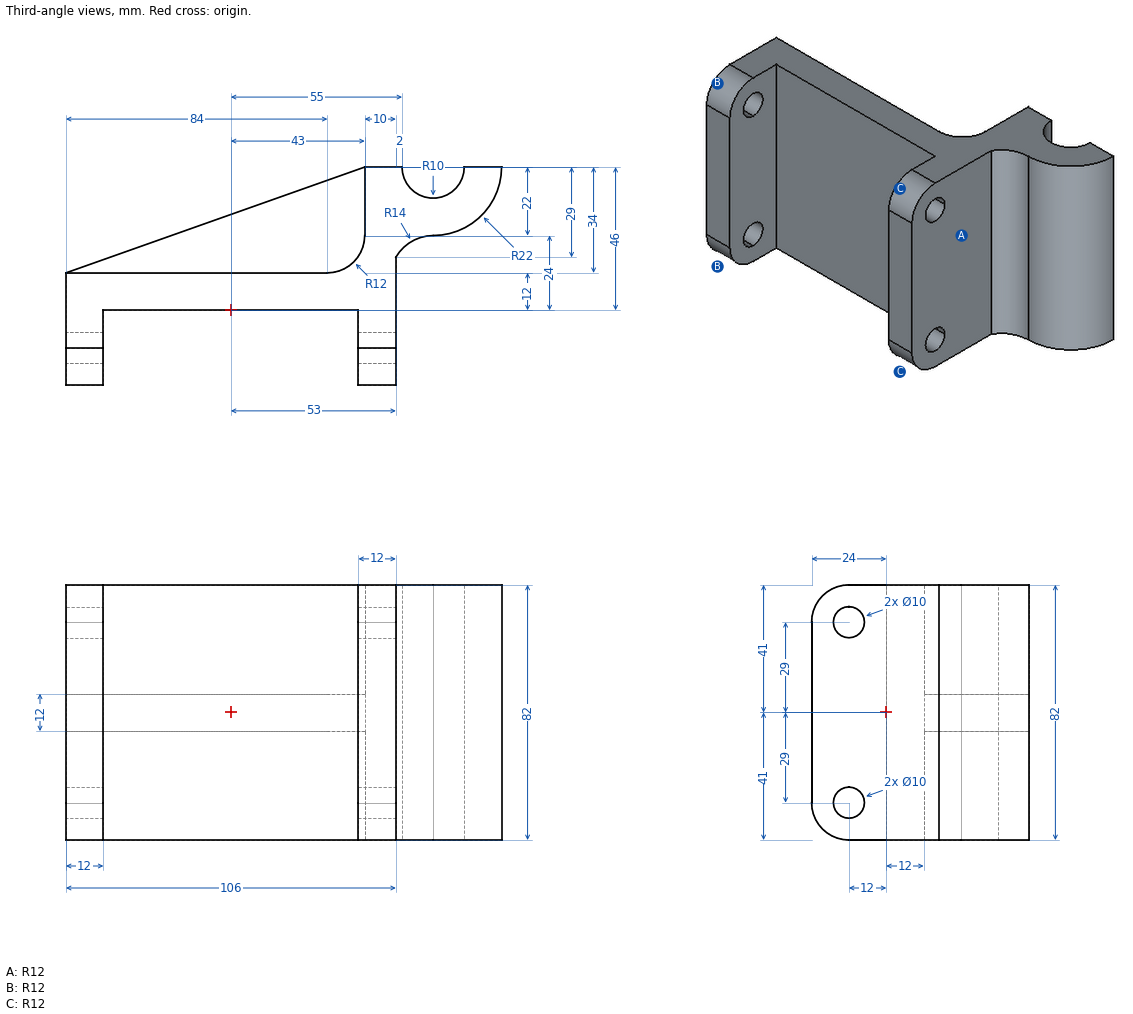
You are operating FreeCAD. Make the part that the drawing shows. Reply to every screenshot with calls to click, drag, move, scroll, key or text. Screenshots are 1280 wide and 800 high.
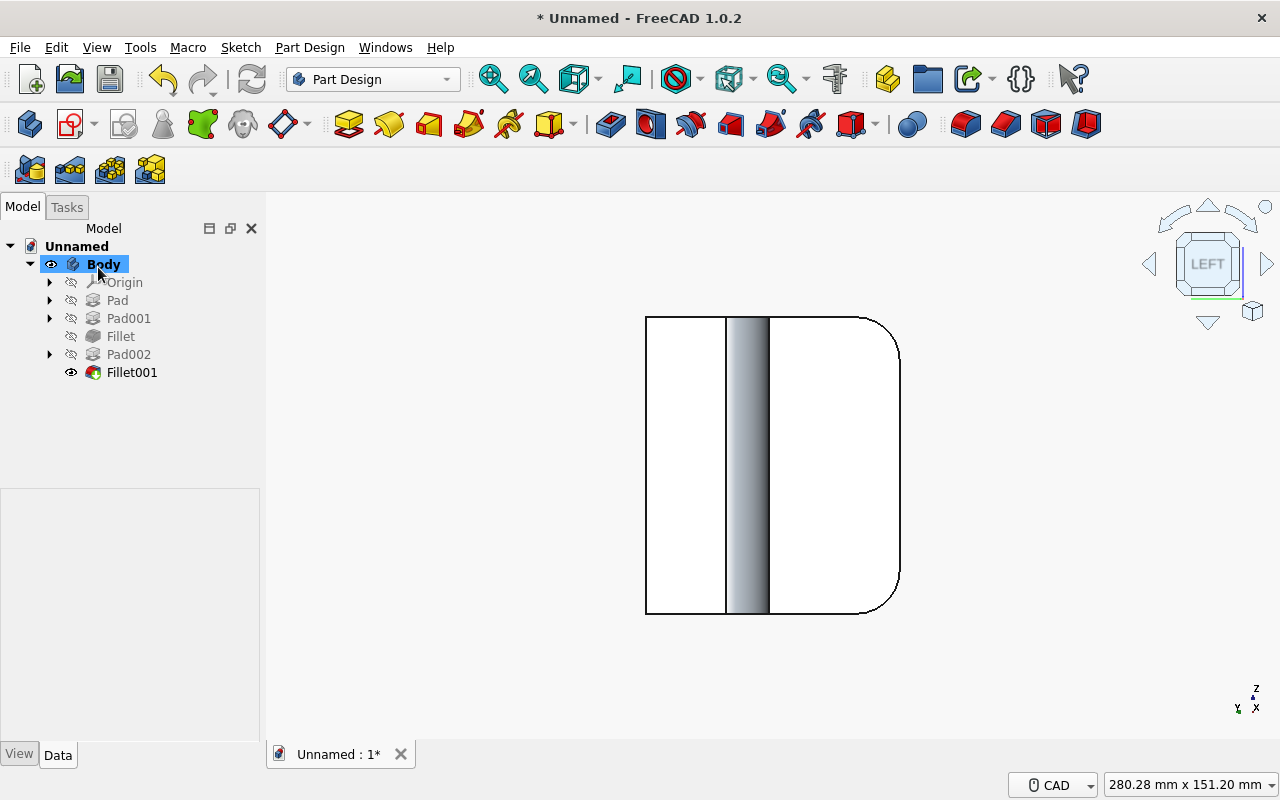
click(835, 422)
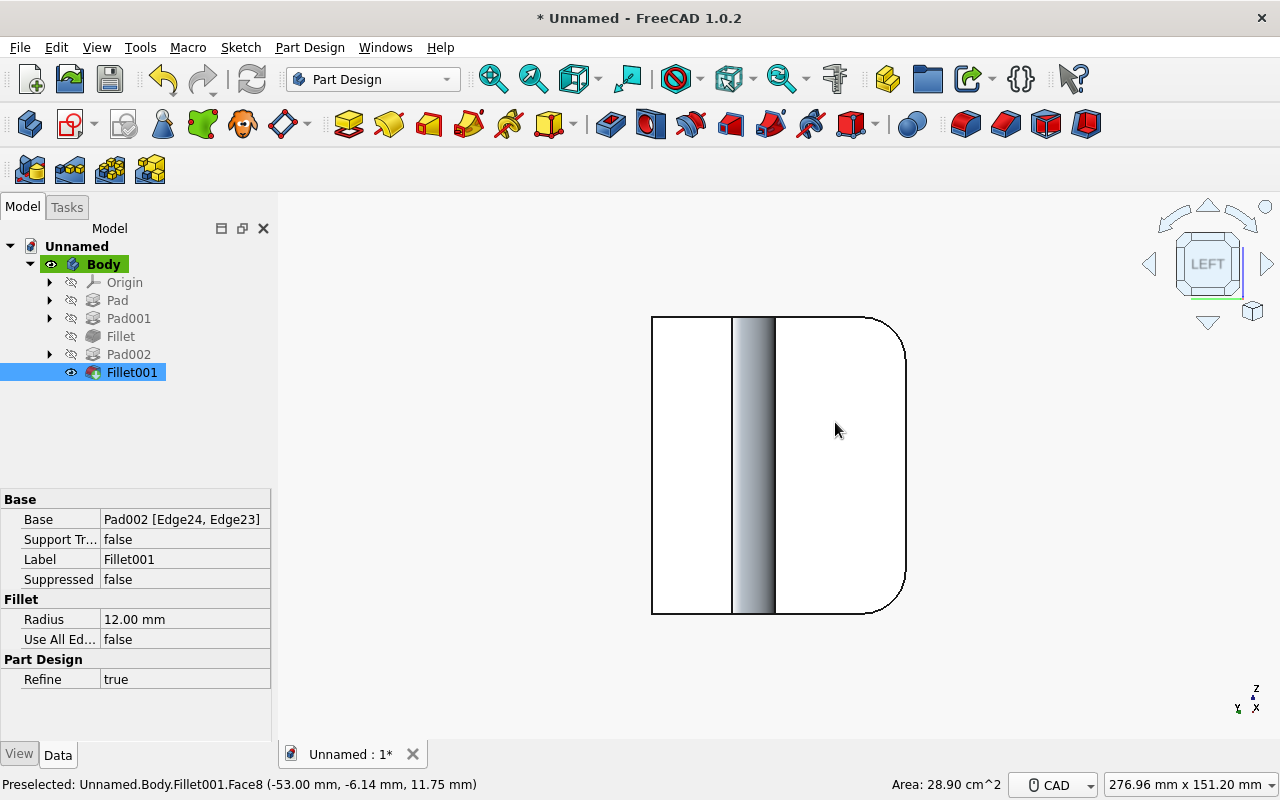
click(70, 124)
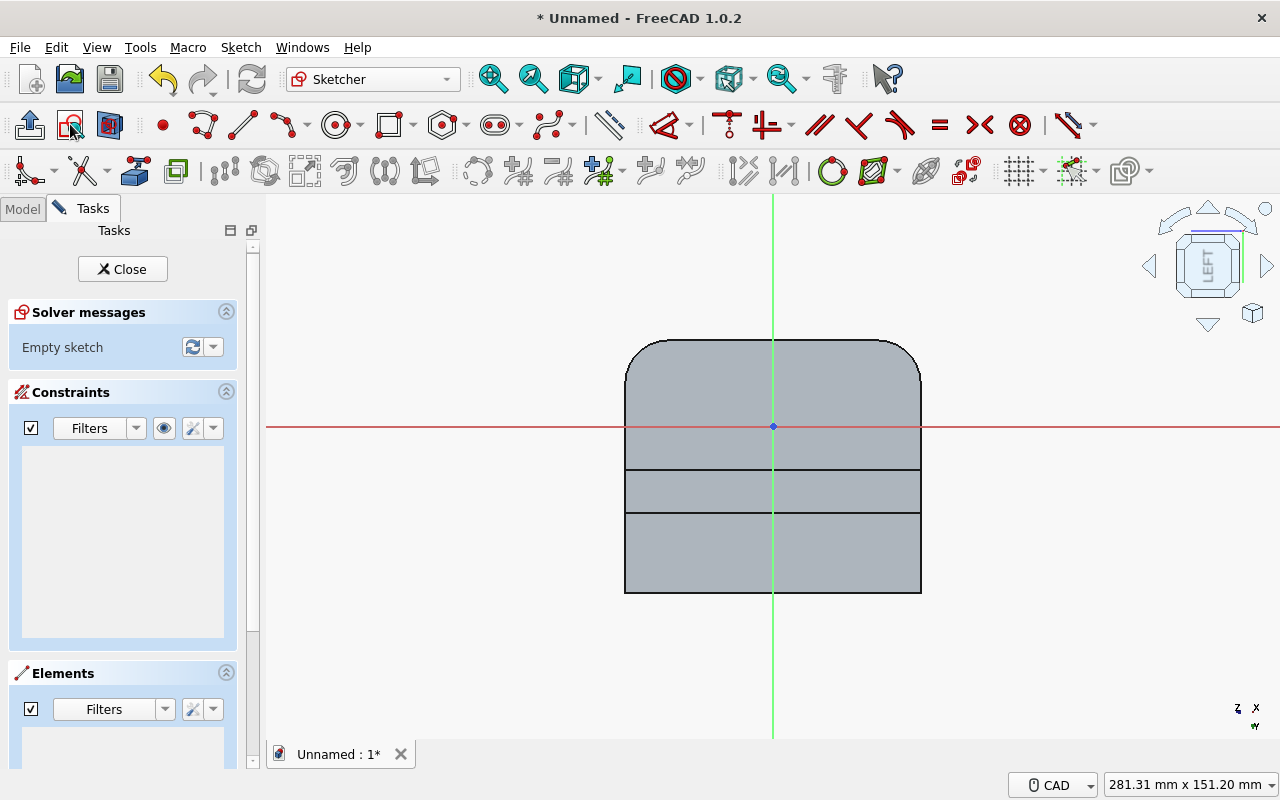
scroll(829, 339, up, 4)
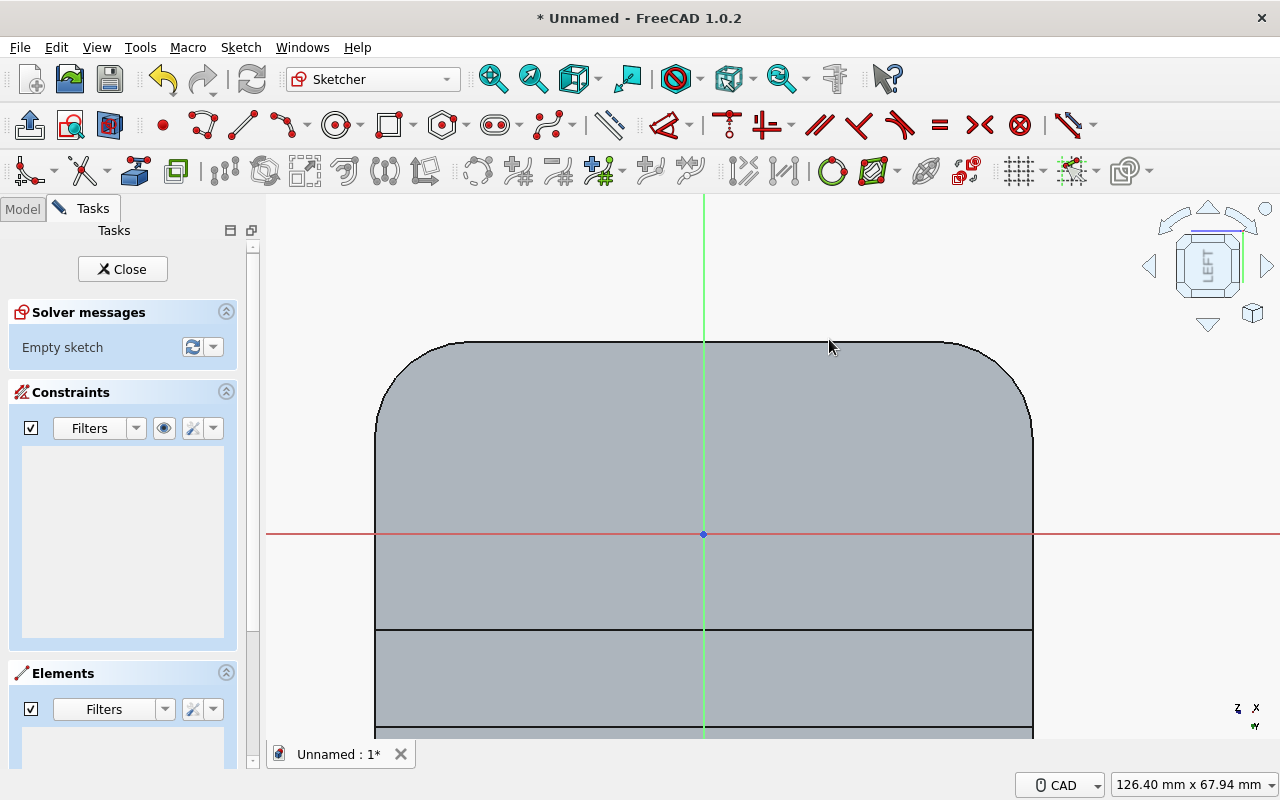
key(g)
key(c)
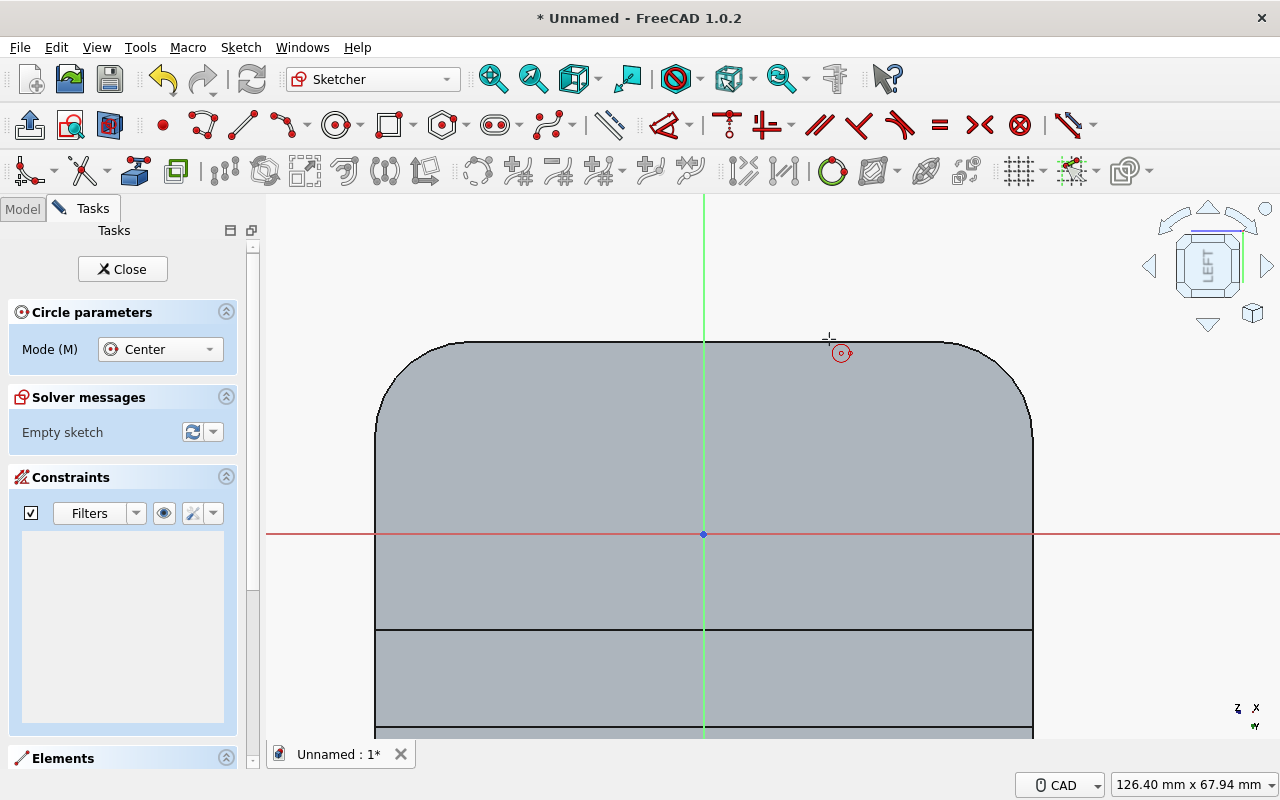
click(936, 438)
move(965, 410)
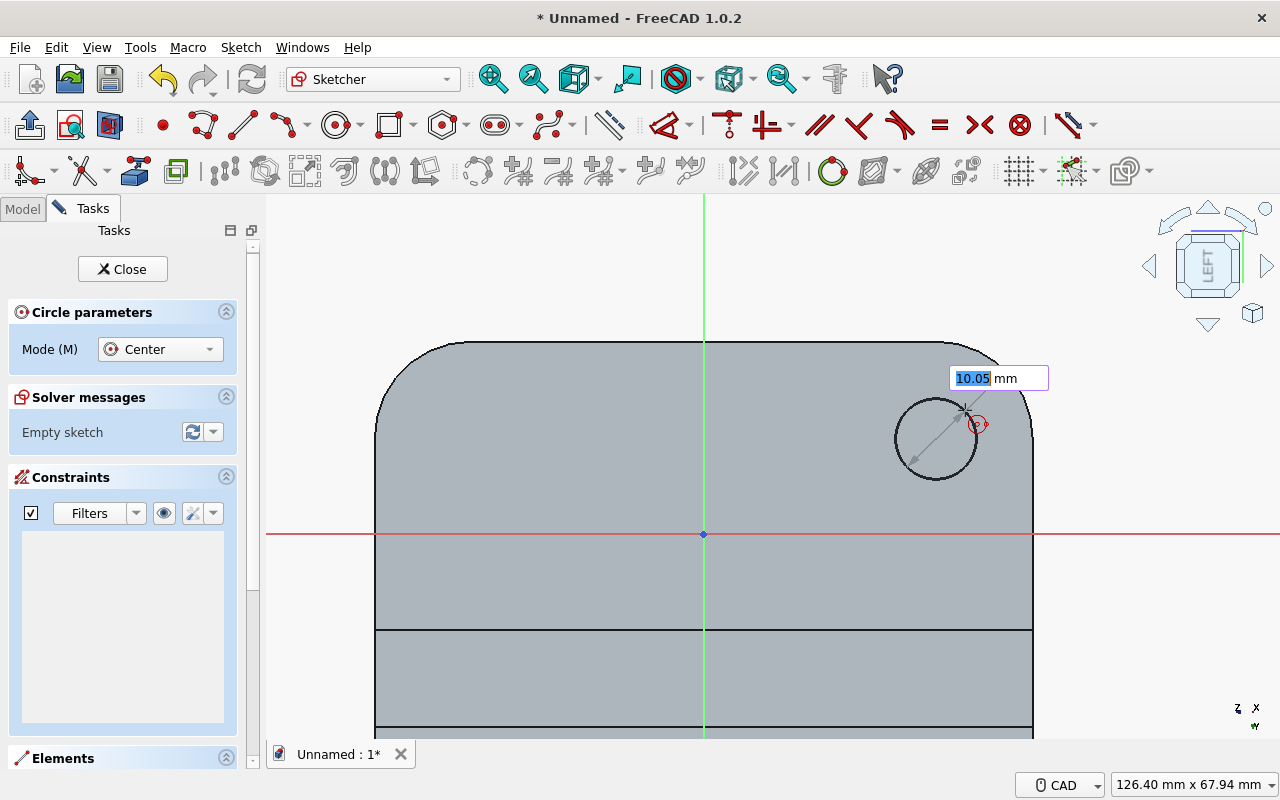
text(10)
key(Return)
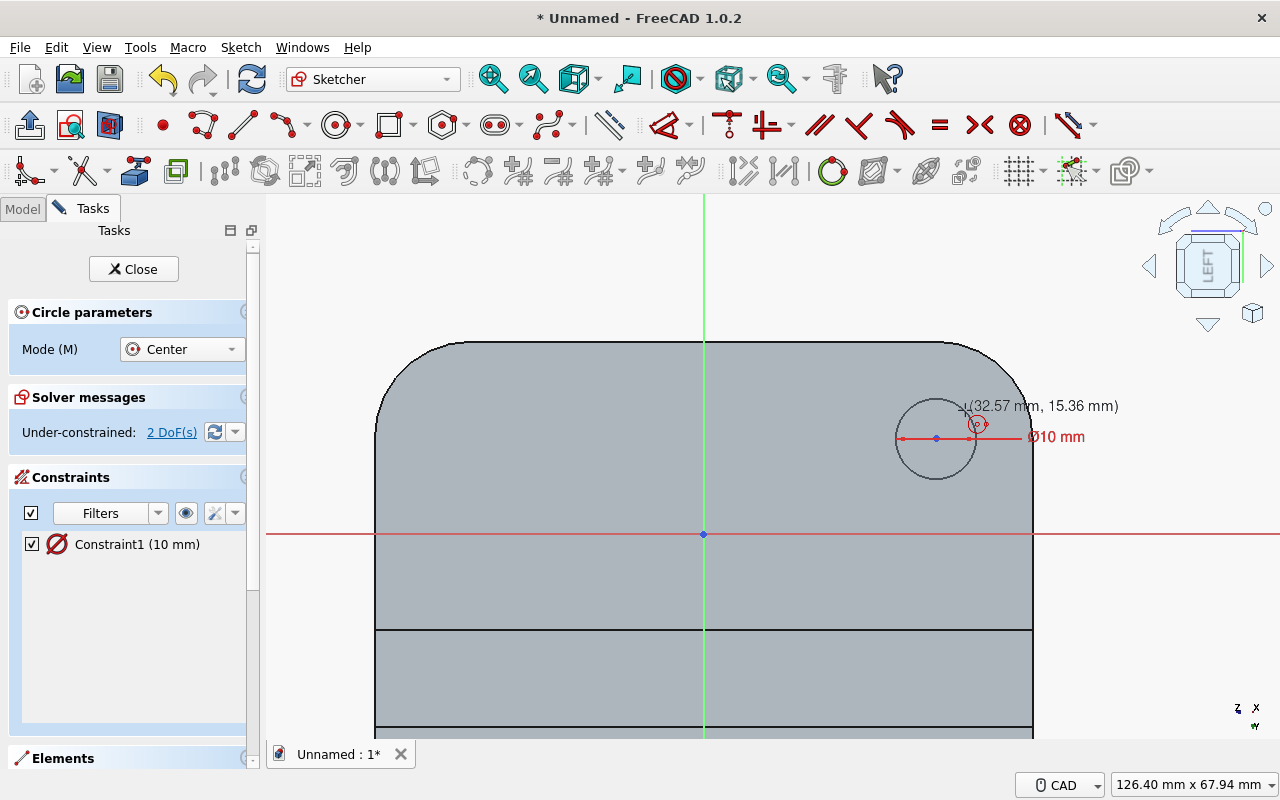
click(471, 438)
move(499, 410)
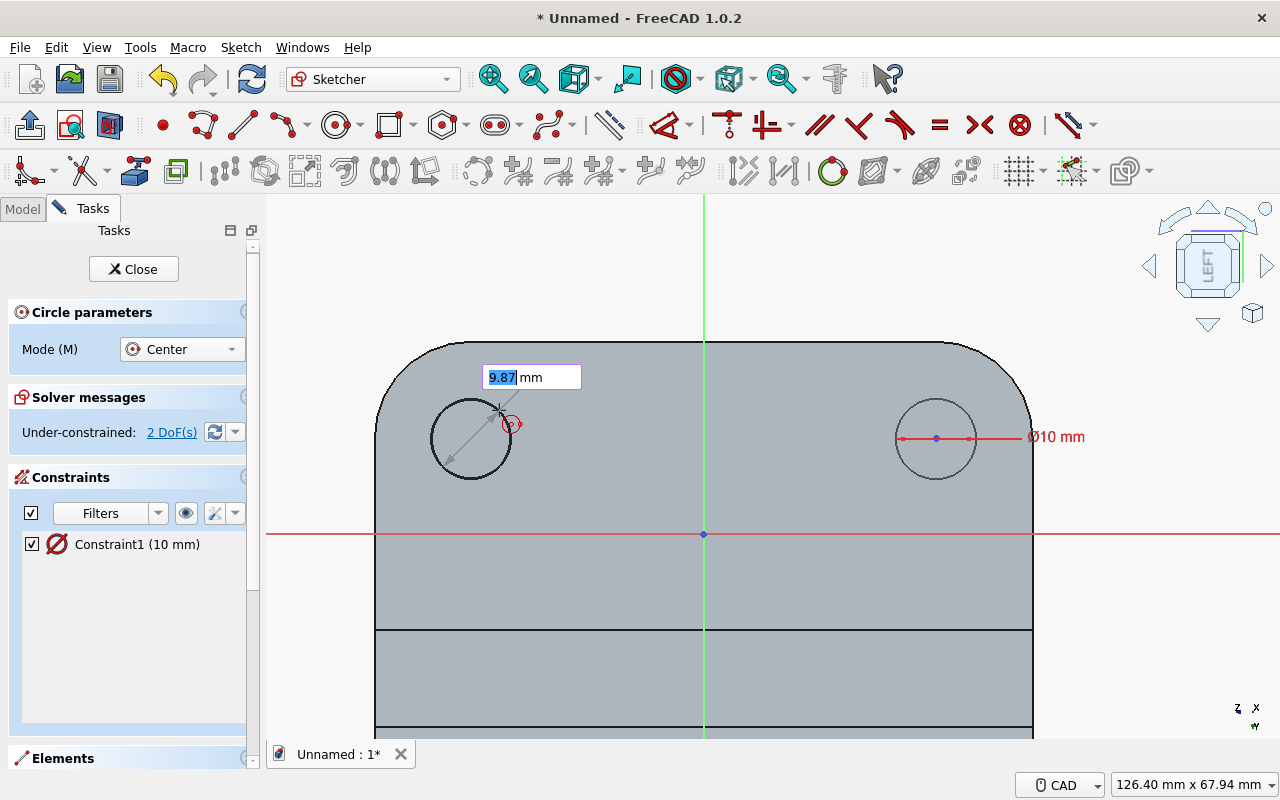
text(10)
key(Return)
key(Escape)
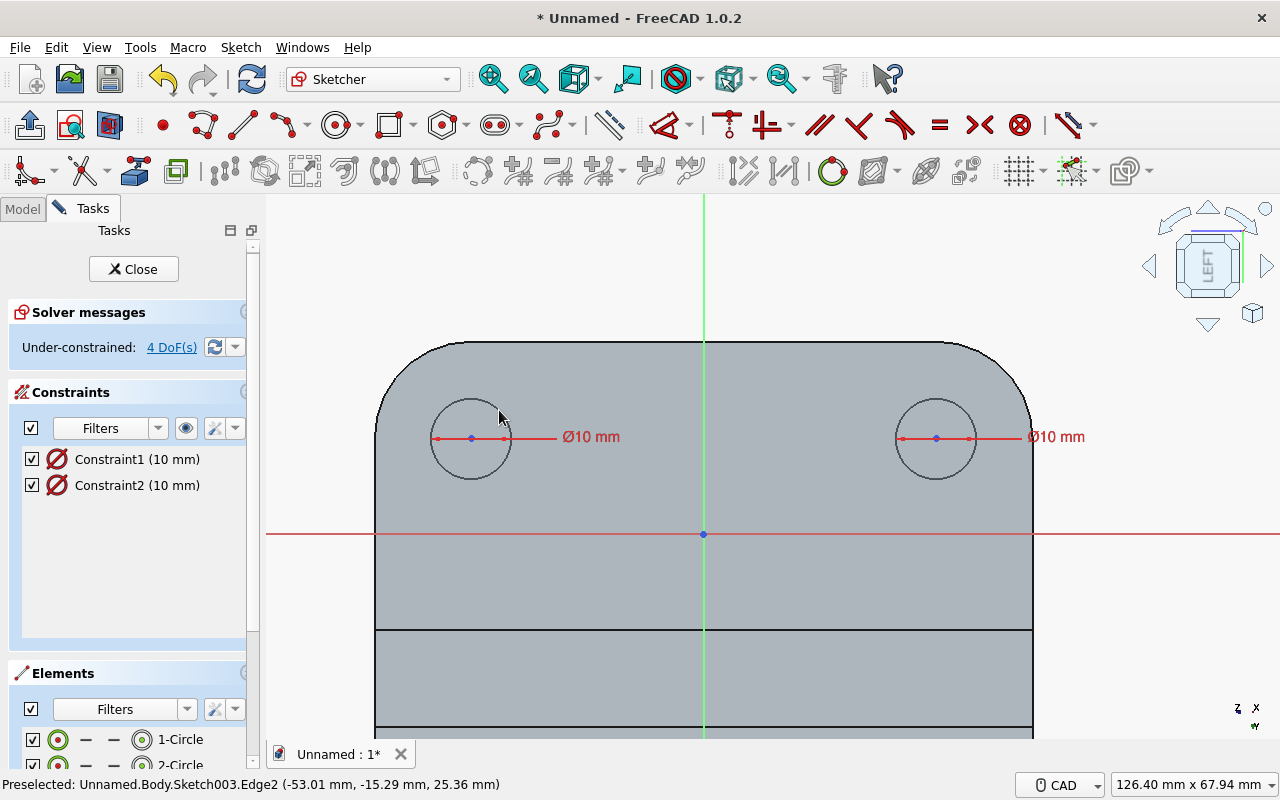
click(936, 439)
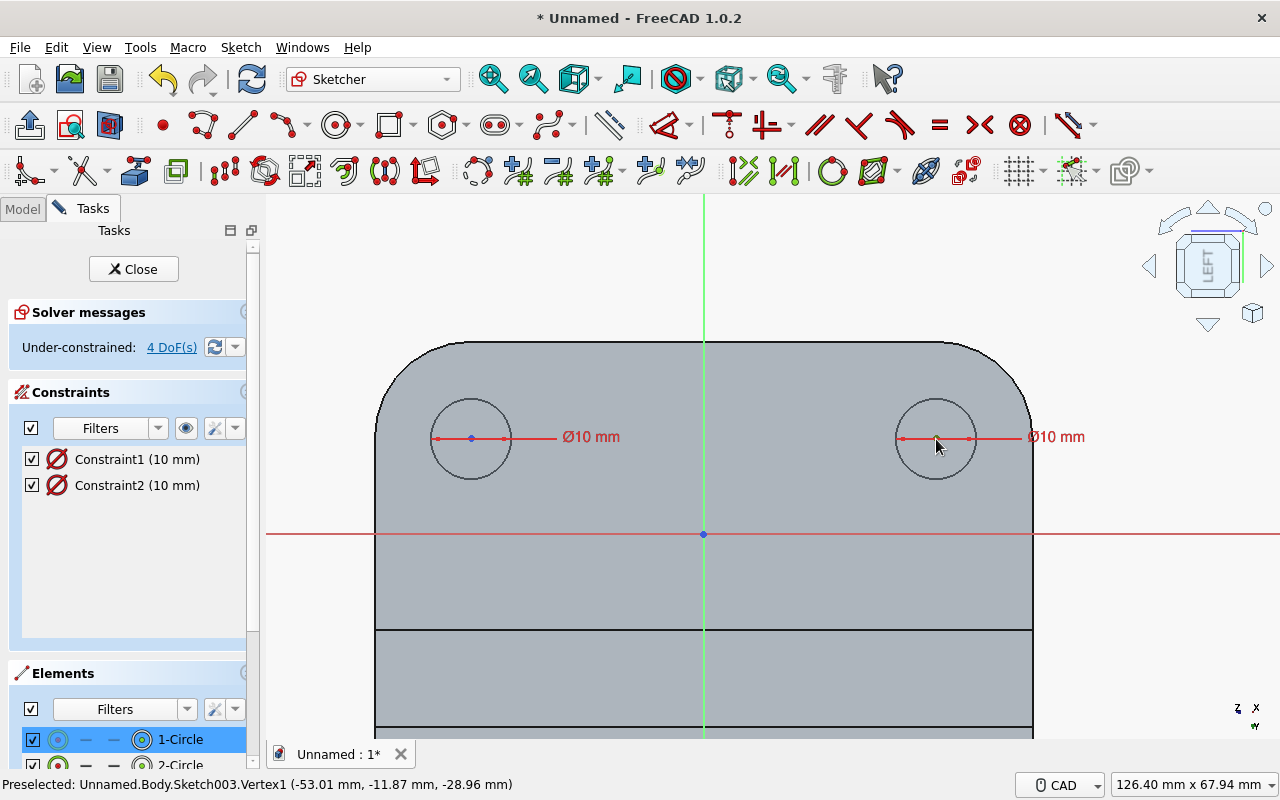
click(471, 439)